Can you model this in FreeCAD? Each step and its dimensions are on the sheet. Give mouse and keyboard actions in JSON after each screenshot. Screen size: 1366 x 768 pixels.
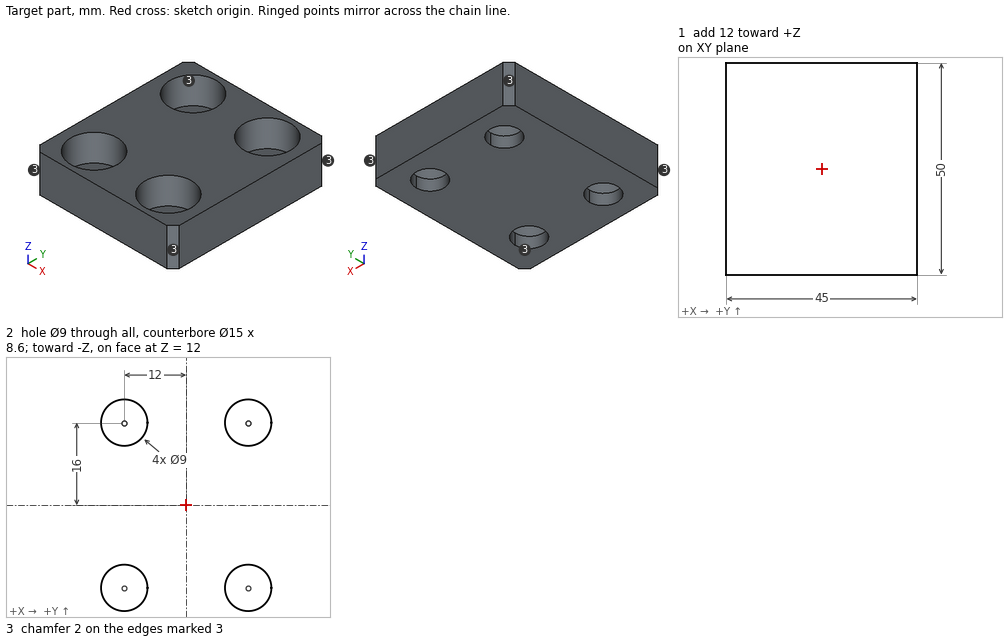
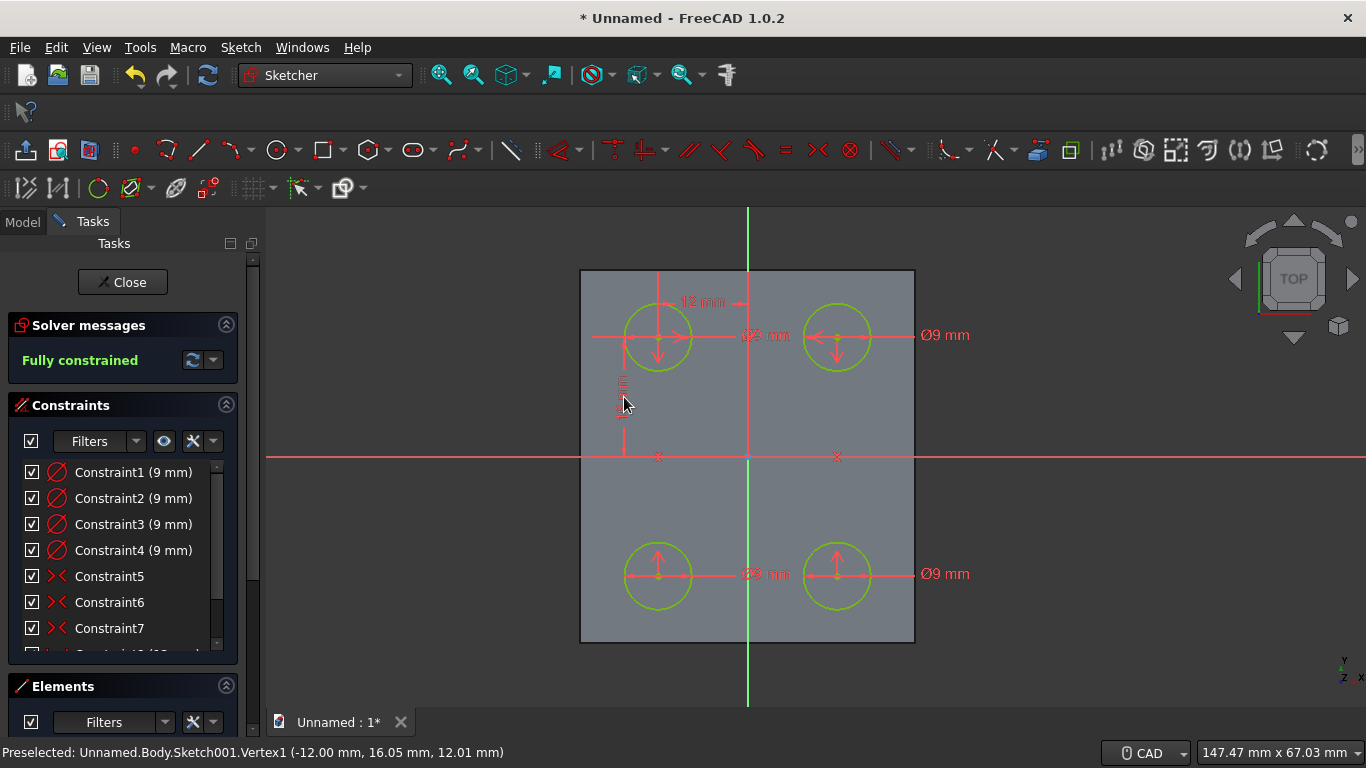
{"action": "left_click", "coordinate": [123, 282]}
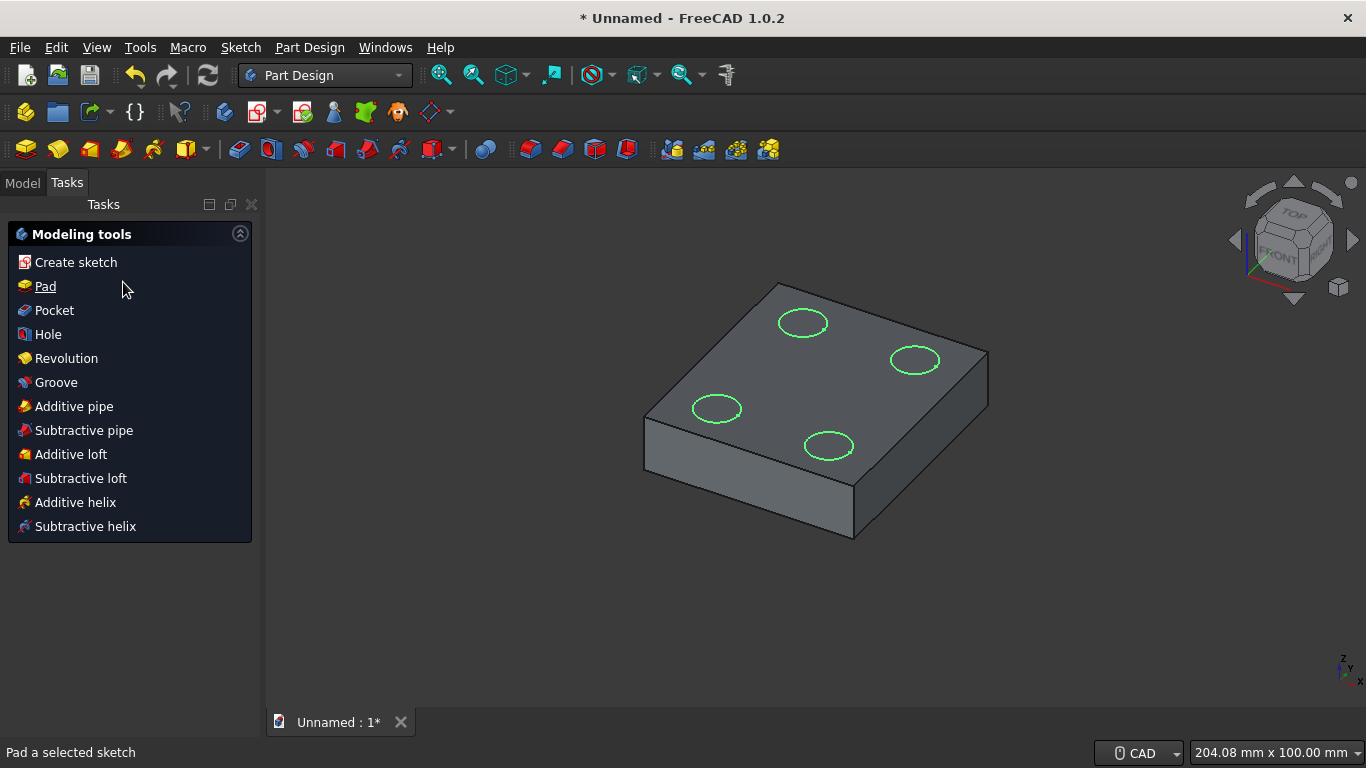
{"action": "left_click", "coordinate": [272, 150]}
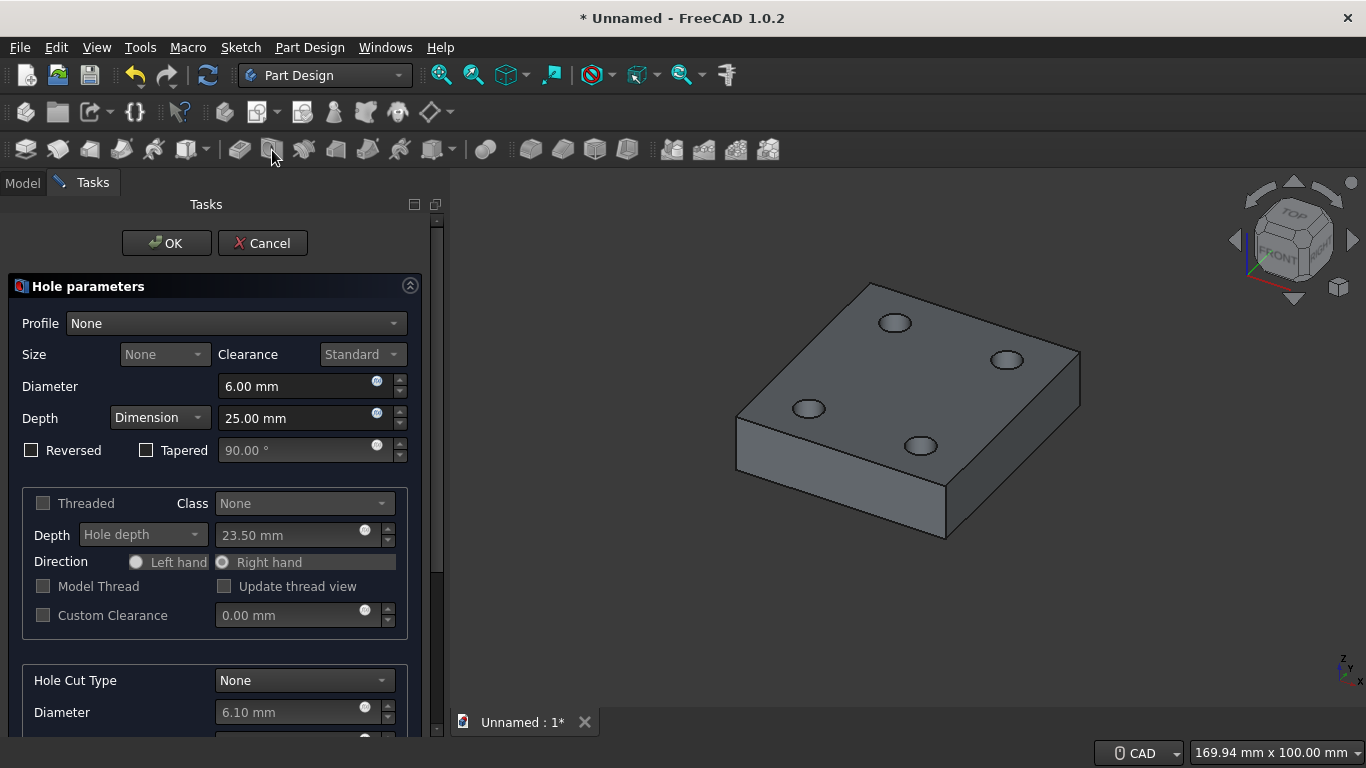
{"action": "triple_click", "coordinate": [305, 386]}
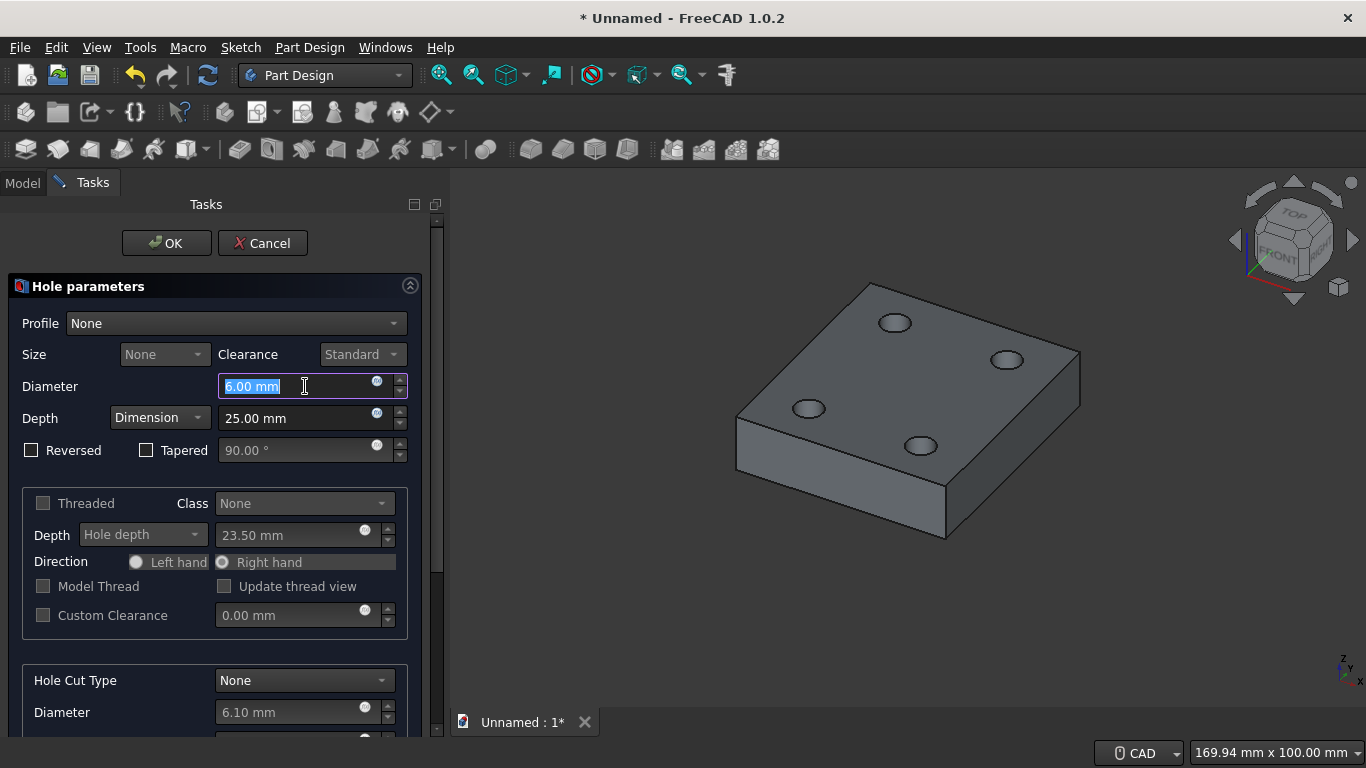
{"action": "type", "text": "9"}
{"action": "key", "text": "Tab"}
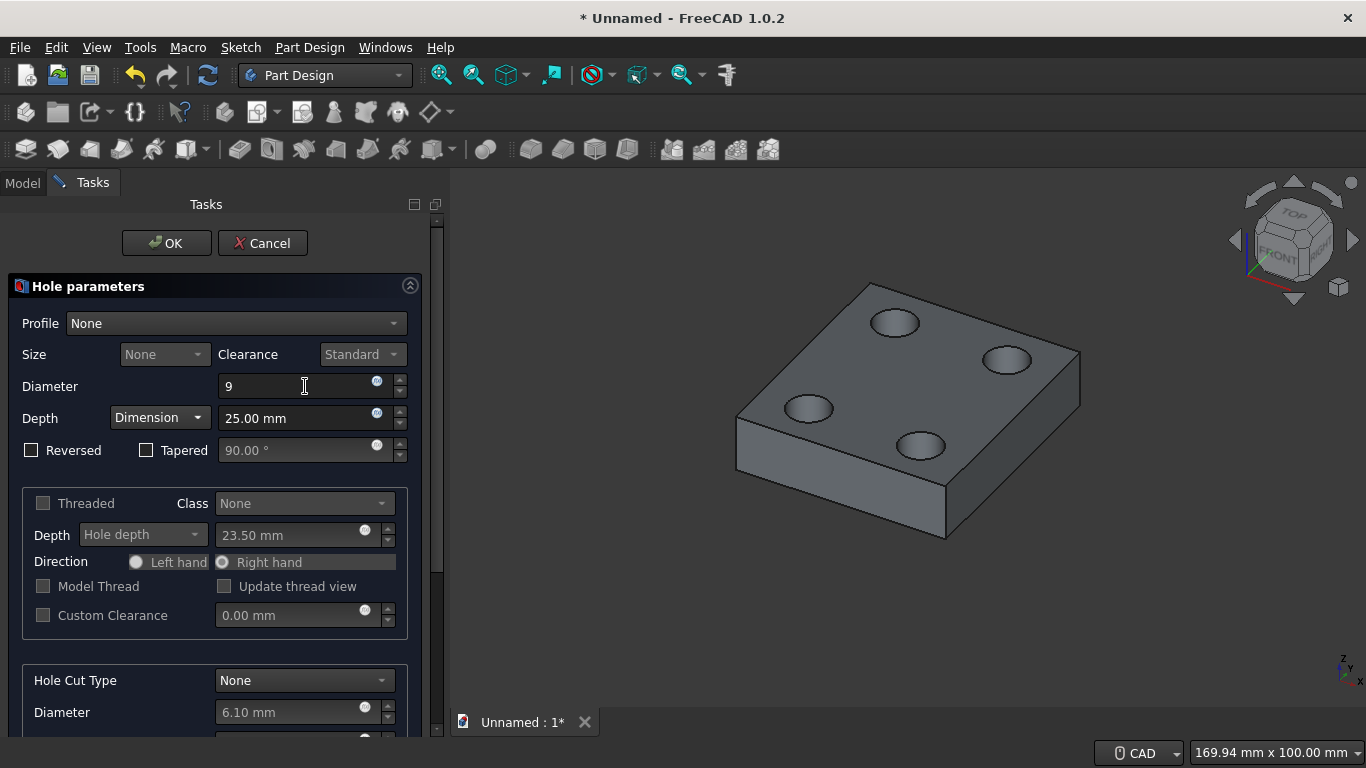
{"action": "left_click", "coordinate": [161, 418]}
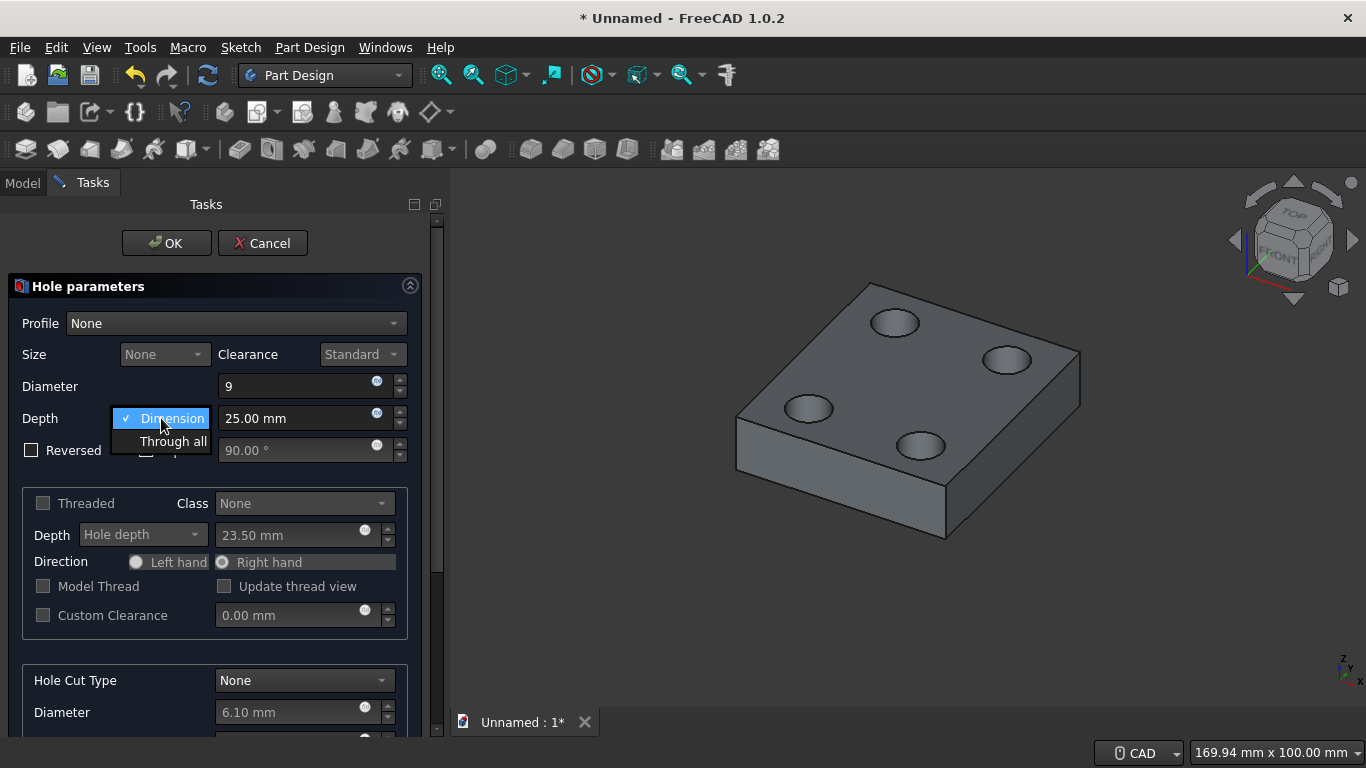
{"action": "left_click", "coordinate": [160, 442]}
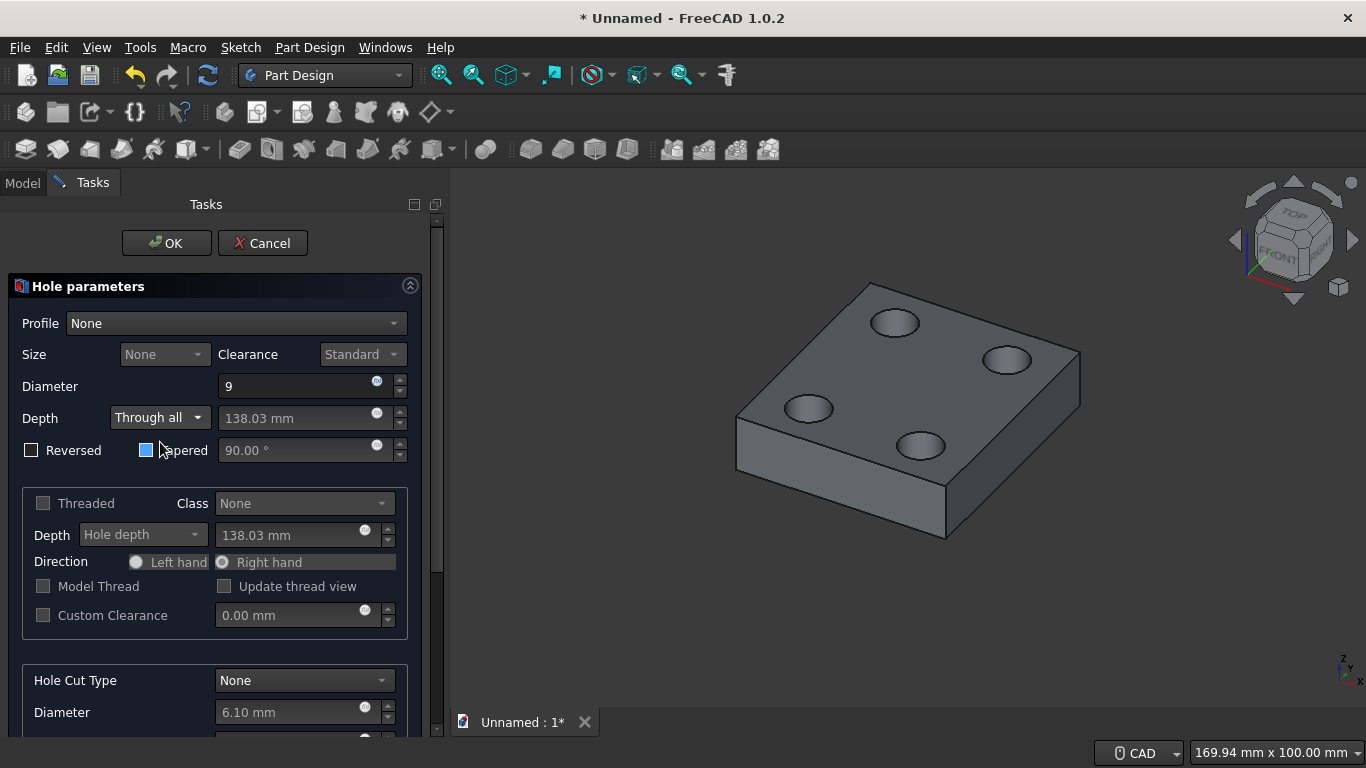
{"action": "left_click", "coordinate": [306, 680]}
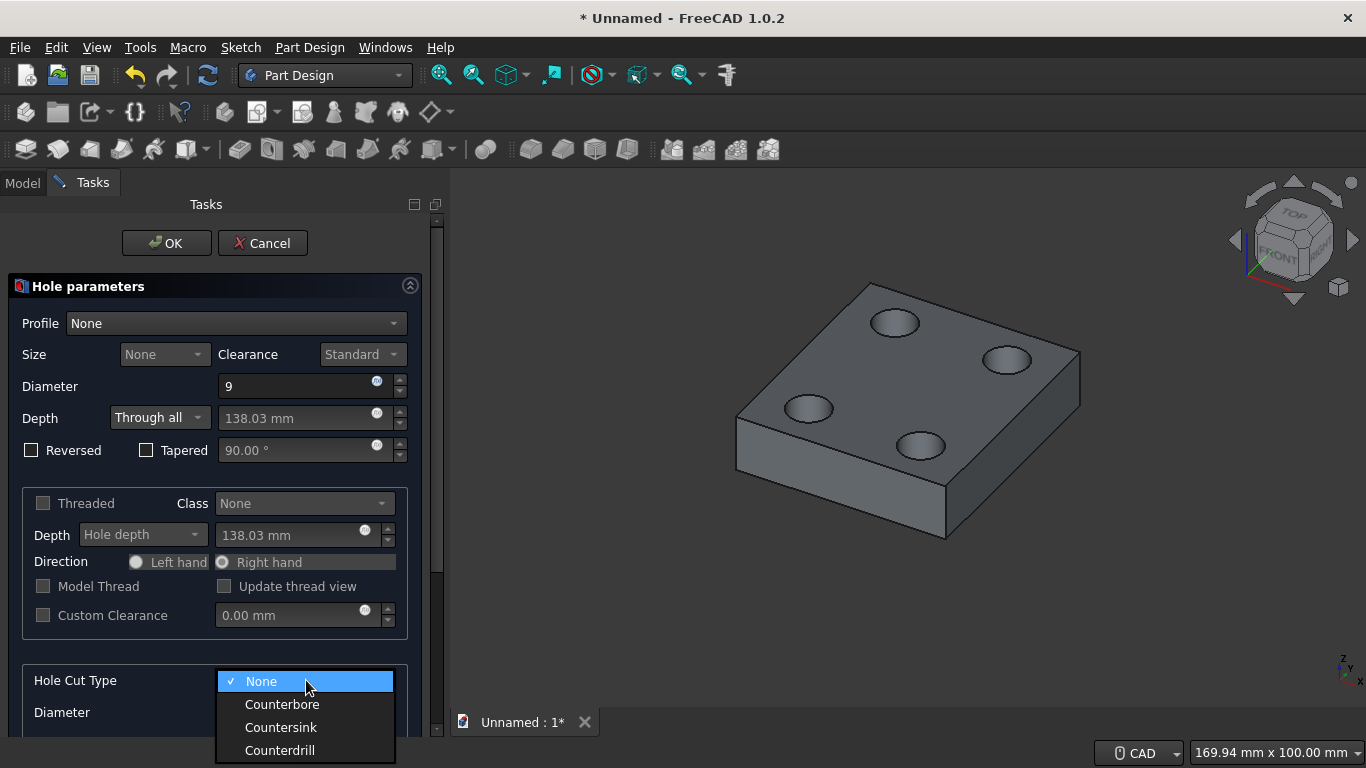
{"action": "left_click", "coordinate": [304, 704]}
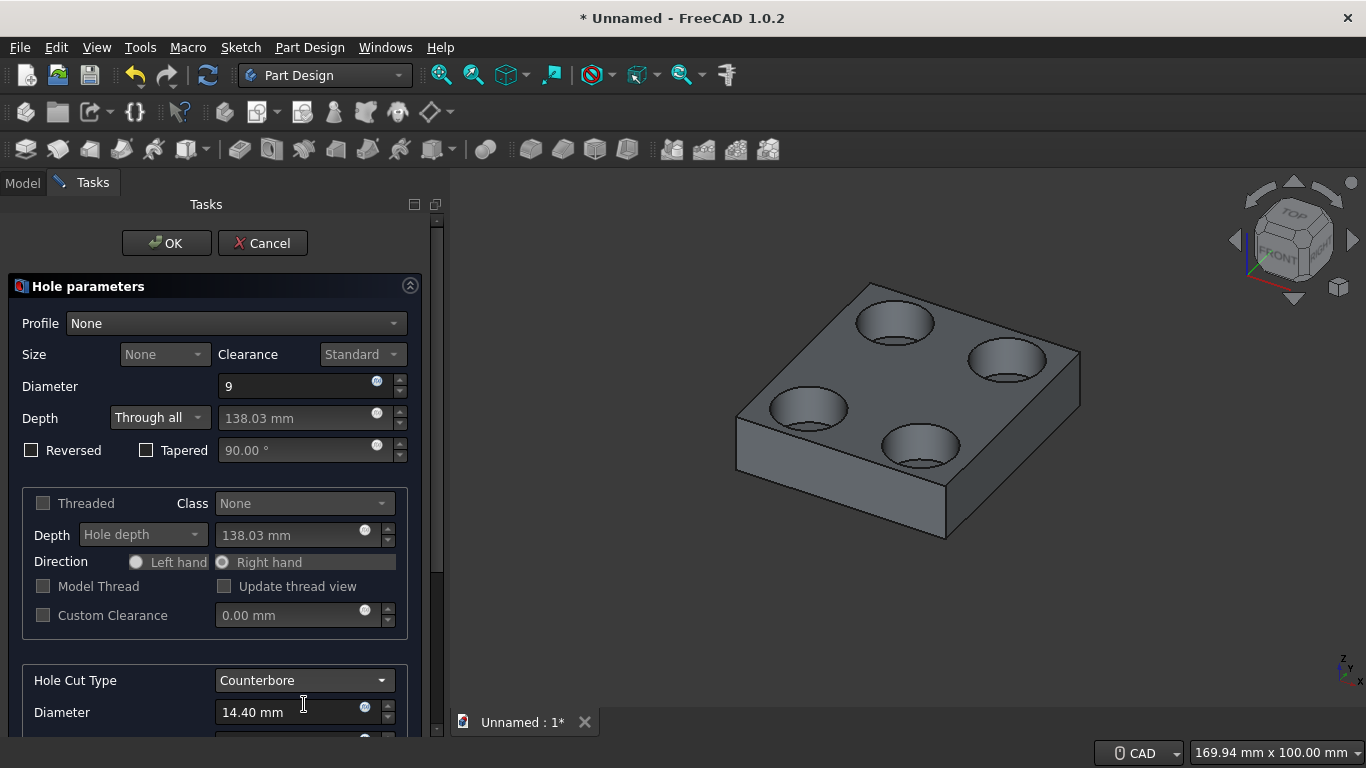
{"action": "triple_click", "coordinate": [298, 712]}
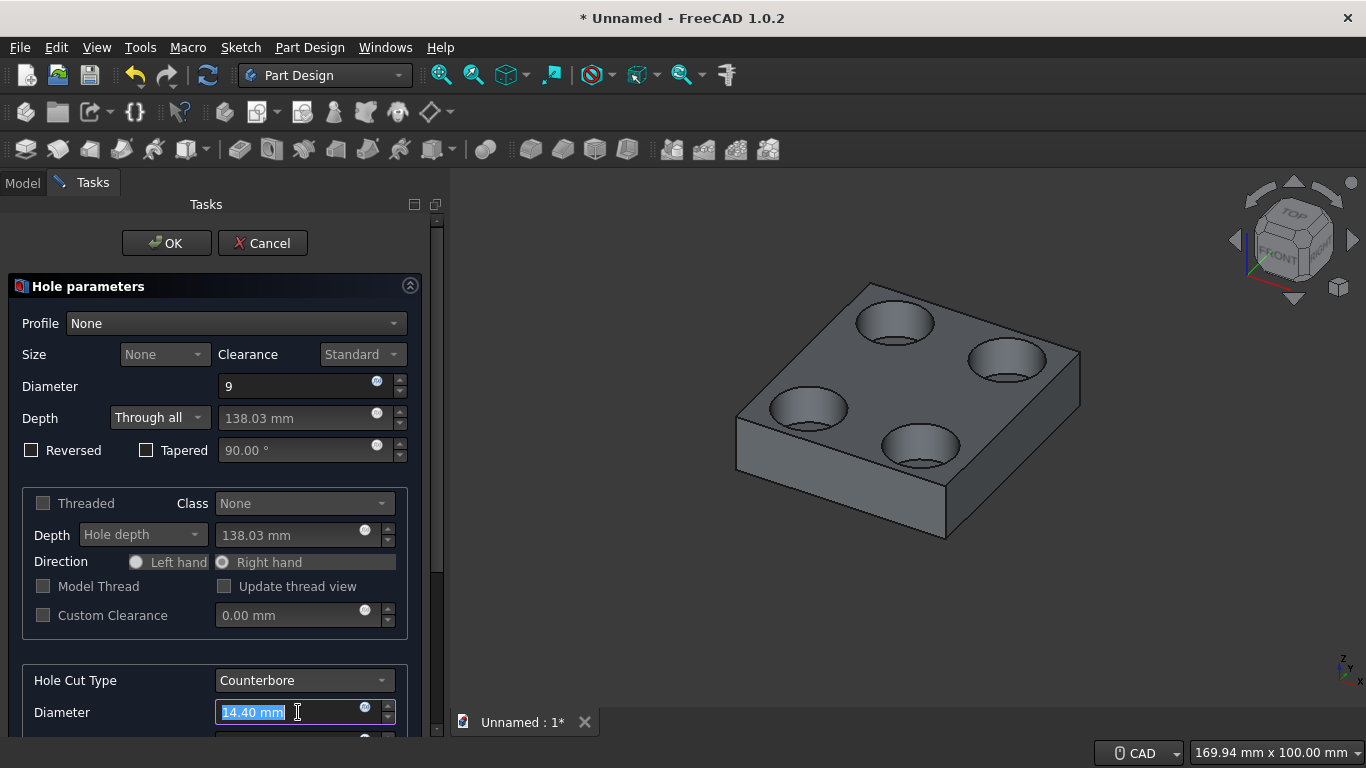
{"action": "type", "text": "15"}
{"action": "key", "text": "Tab"}